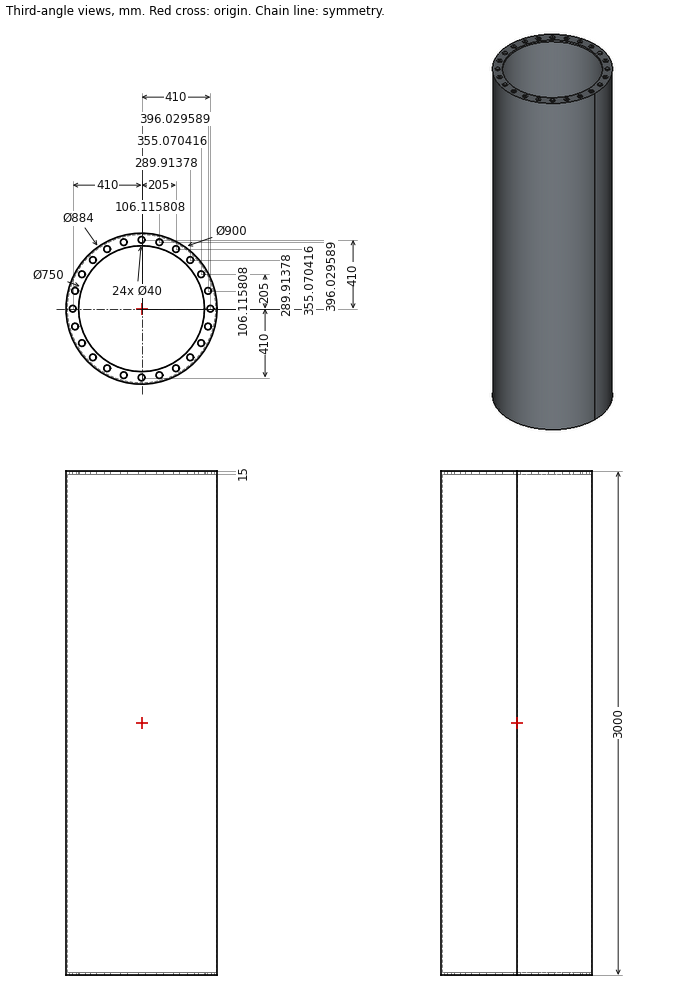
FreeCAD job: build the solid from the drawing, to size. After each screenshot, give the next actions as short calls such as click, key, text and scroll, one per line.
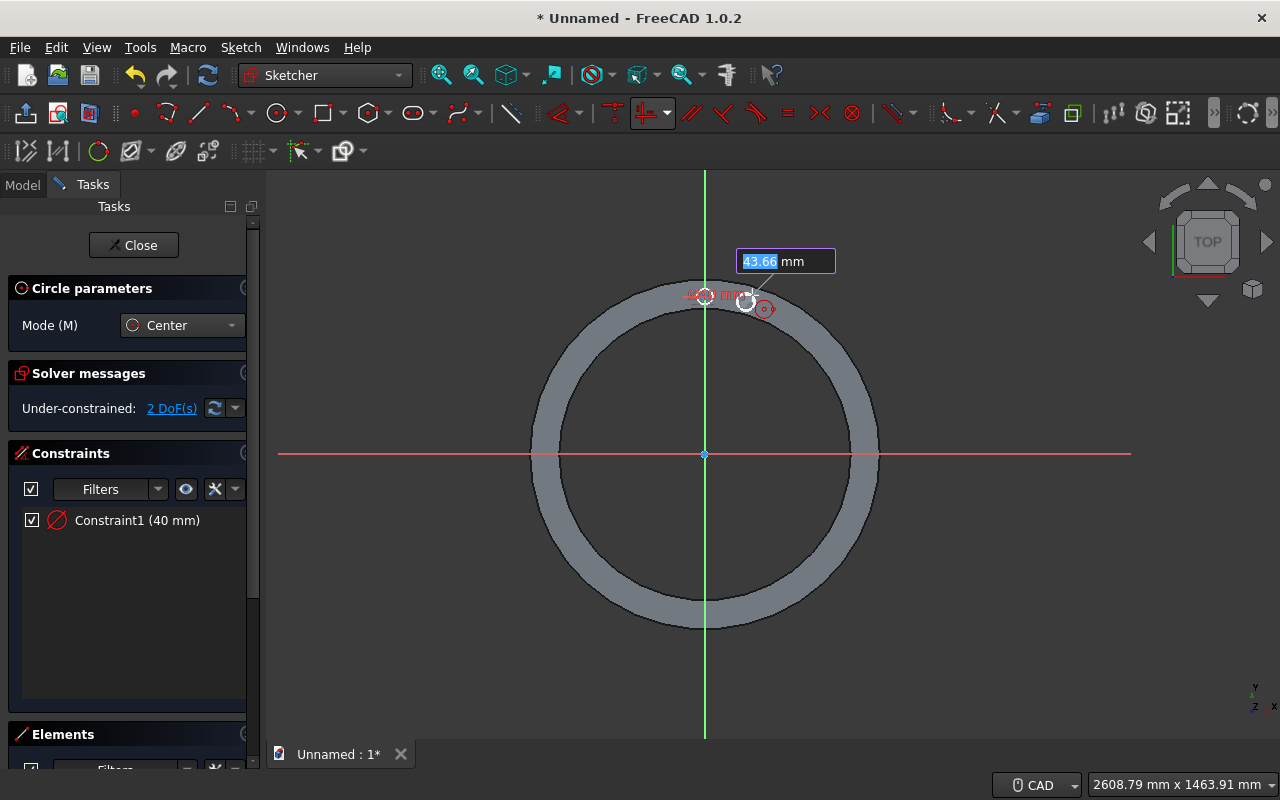
text(40)
key(Return)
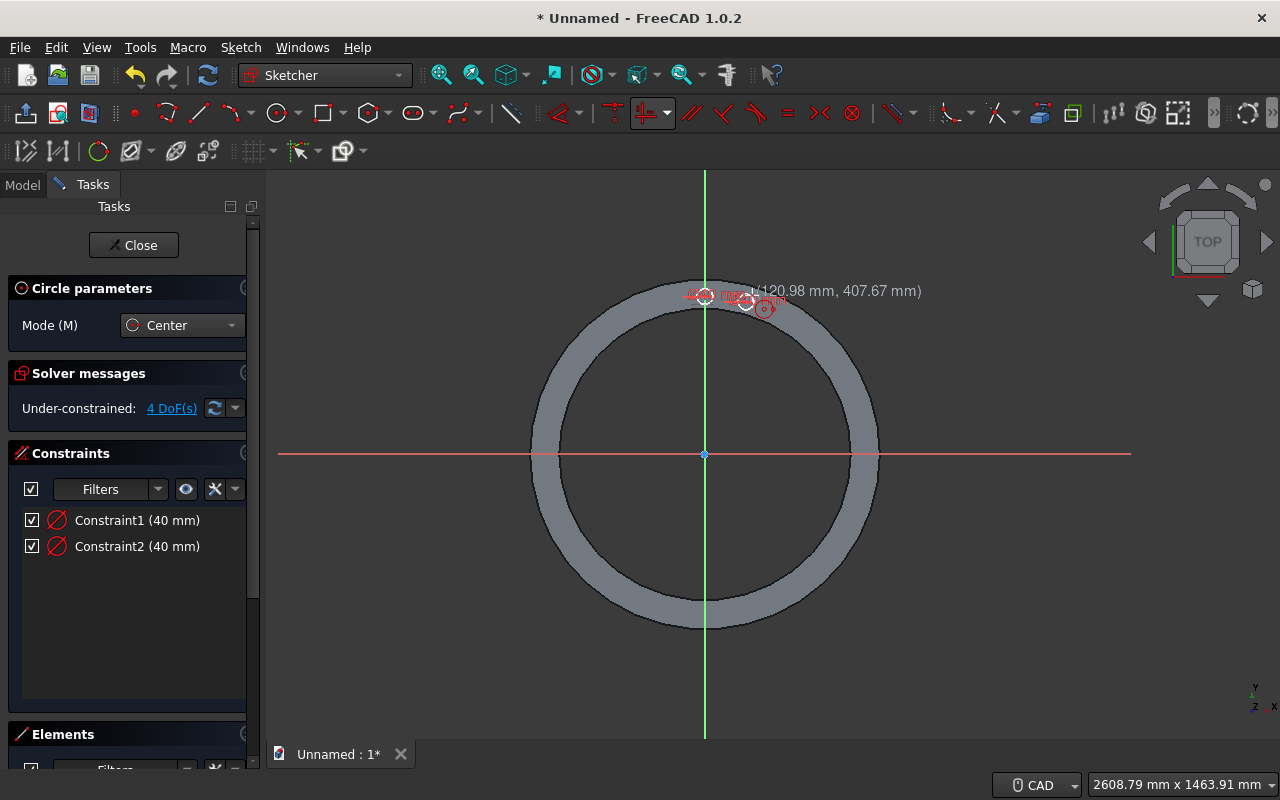
scroll(785, 316, up, 6)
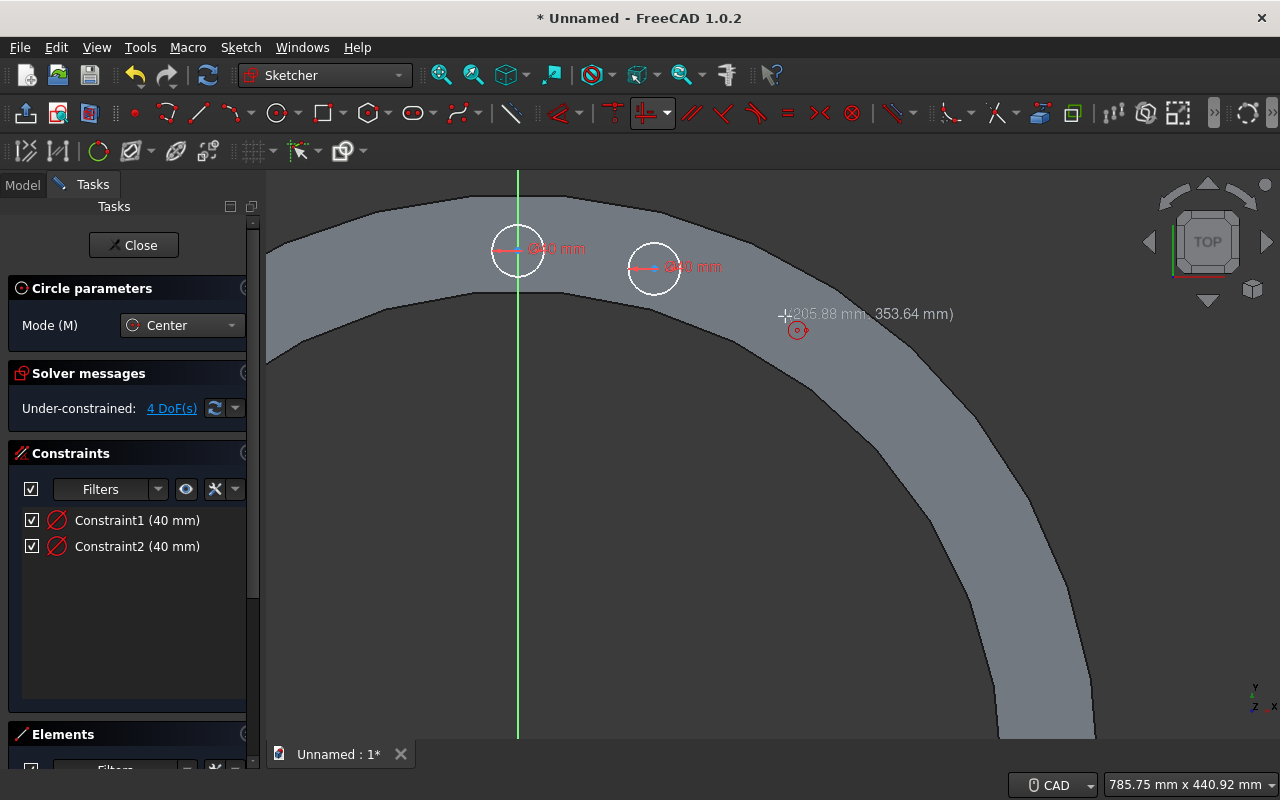
scroll(785, 316, down, 6)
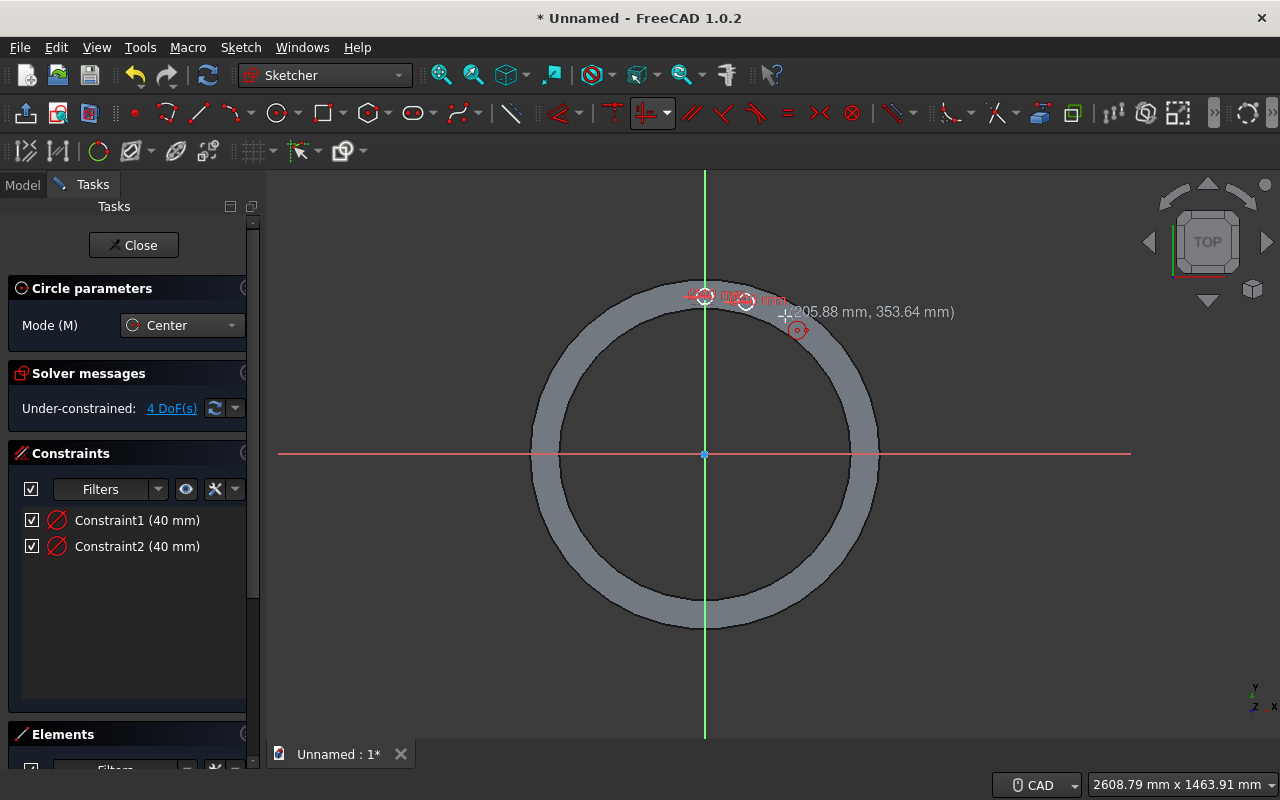
click(785, 316)
move(790, 311)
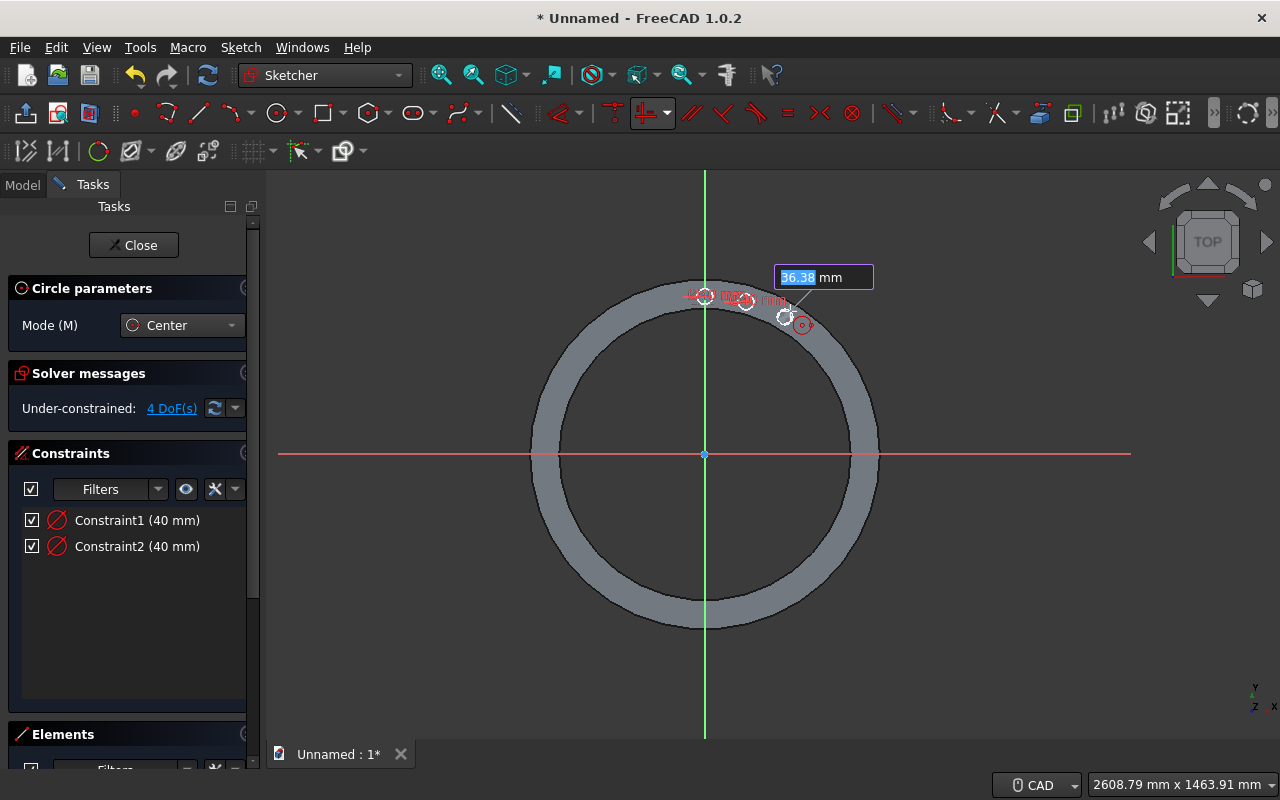
text(40)
key(Return)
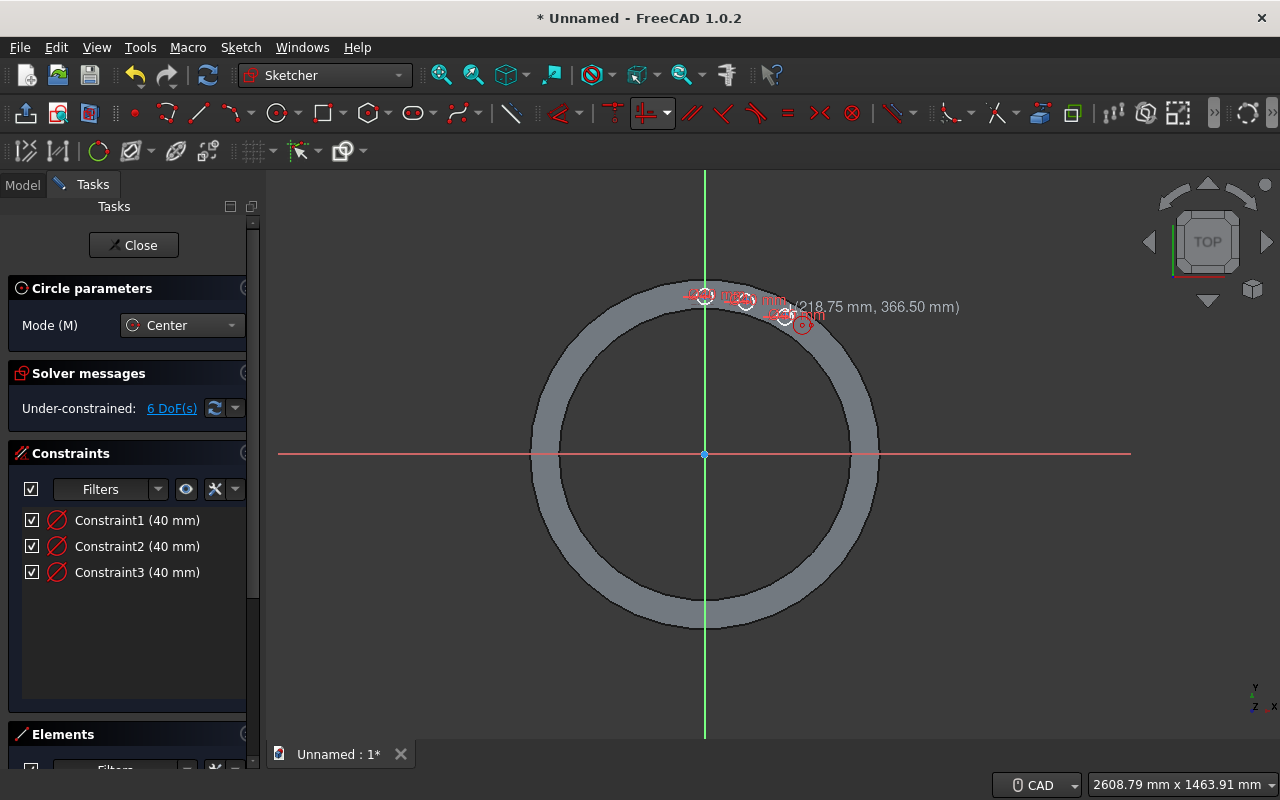
scroll(818, 342, up, 6)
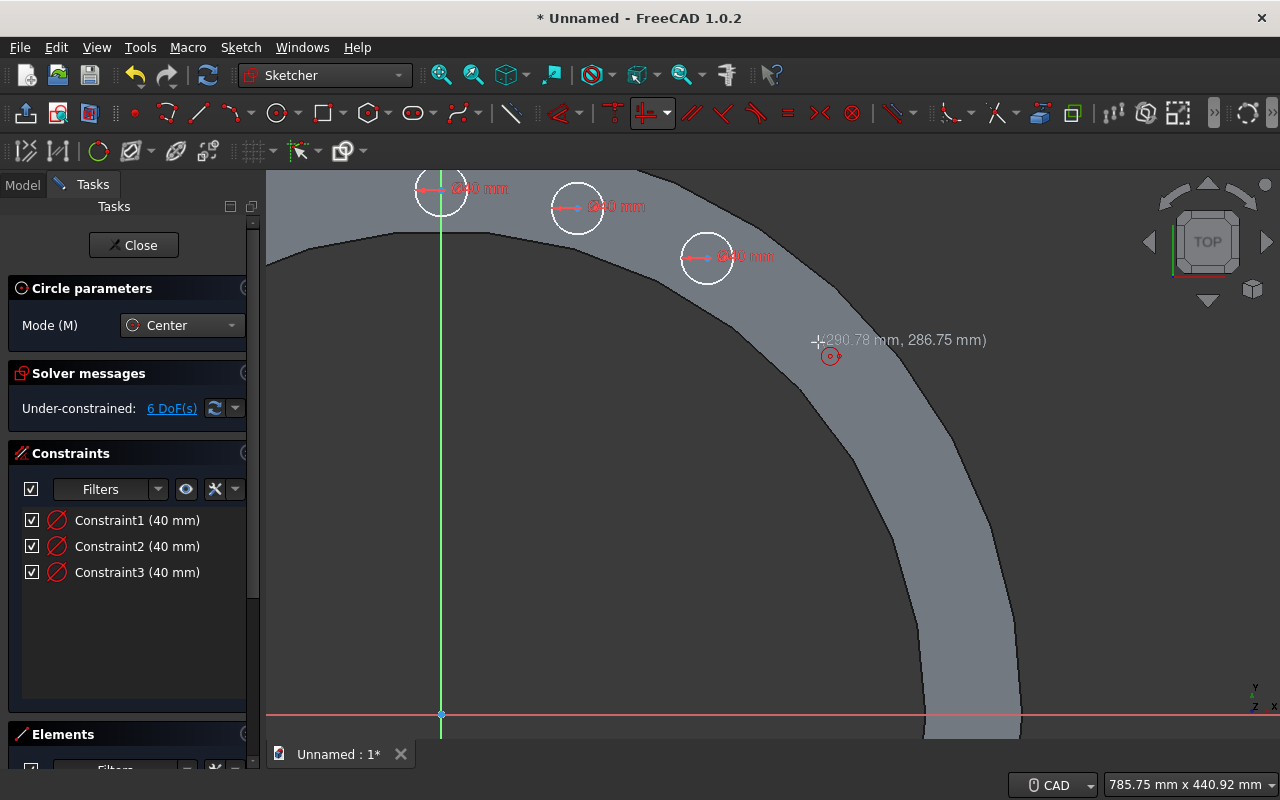
scroll(818, 342, down, 6)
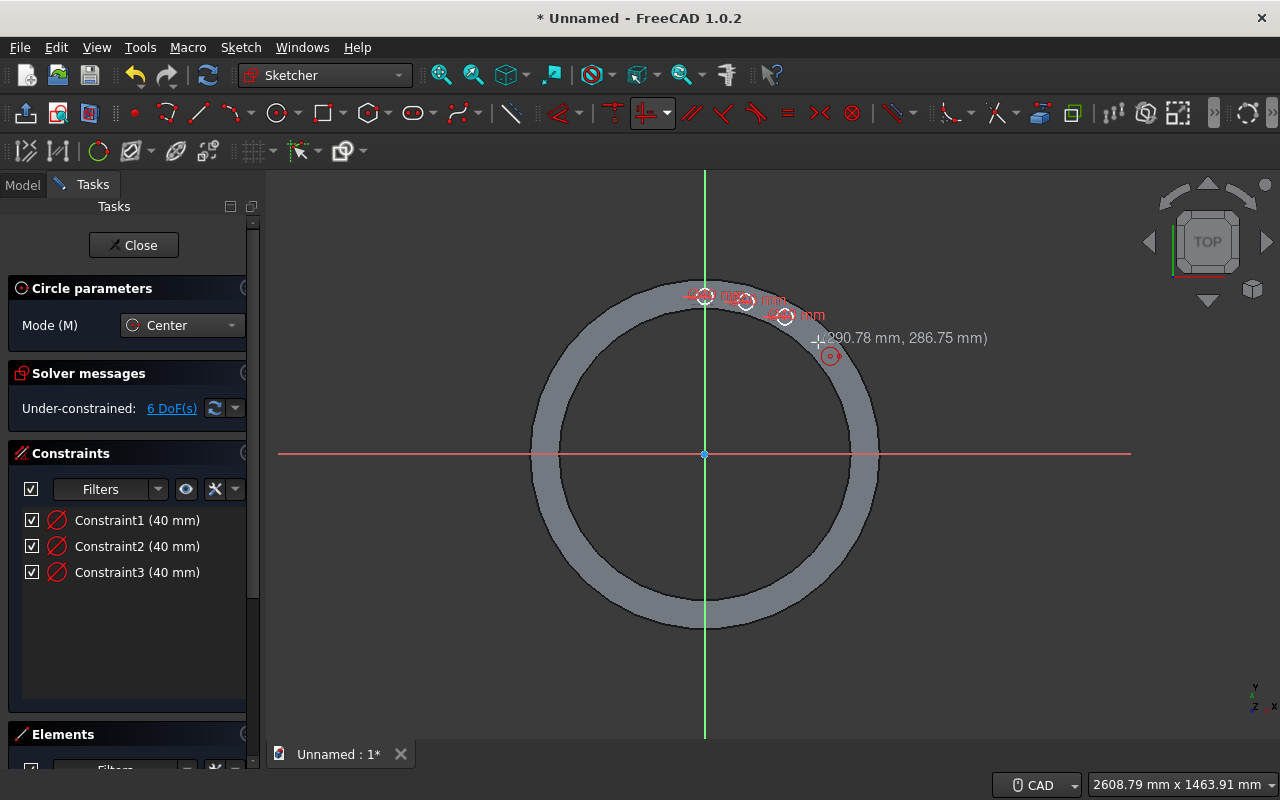
click(818, 342)
move(823, 336)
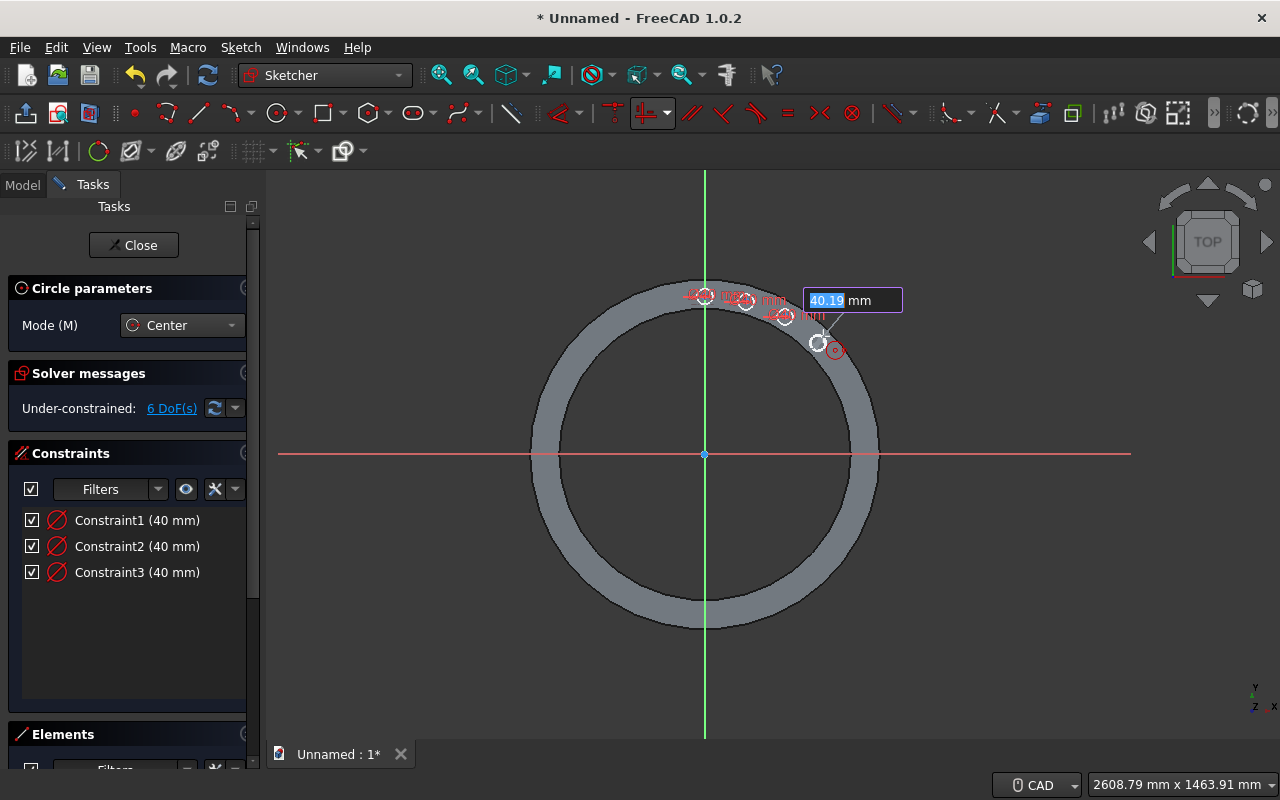
text(40)
key(Return)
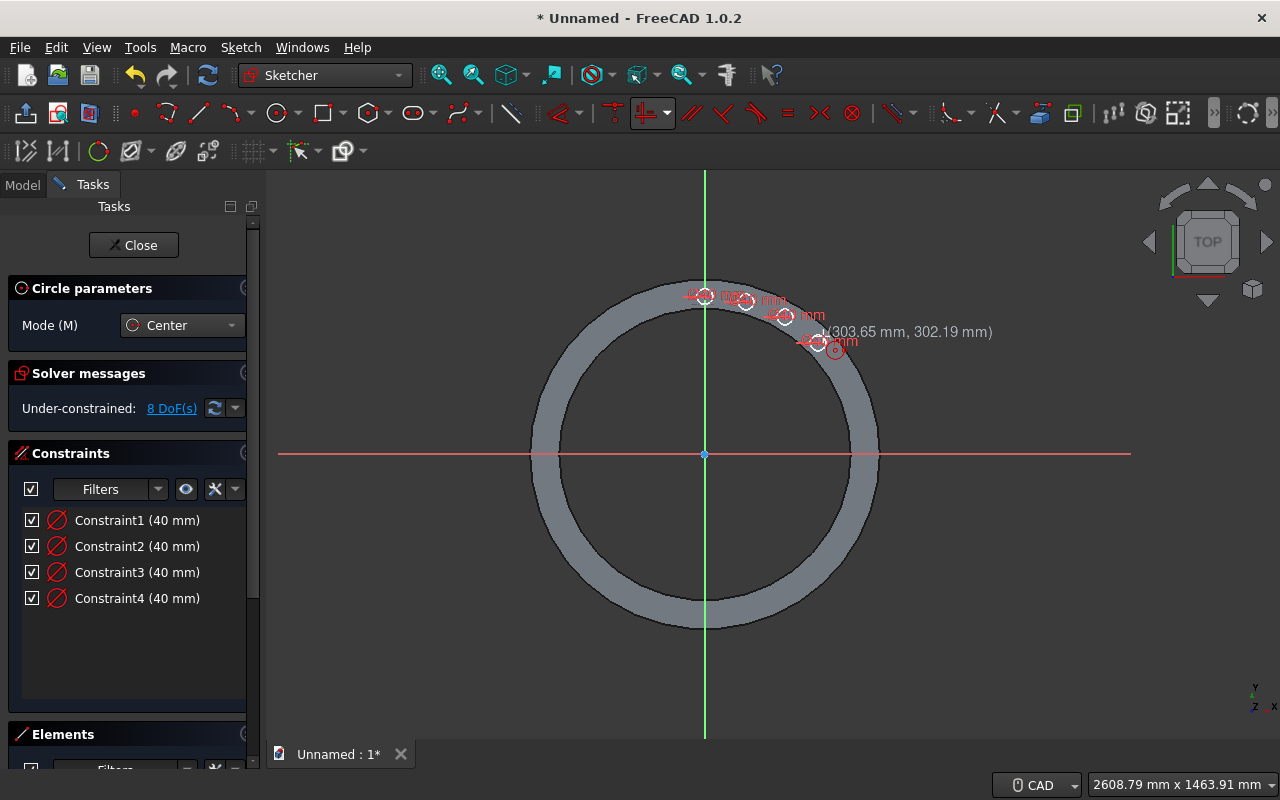
scroll(843, 375, up, 6)